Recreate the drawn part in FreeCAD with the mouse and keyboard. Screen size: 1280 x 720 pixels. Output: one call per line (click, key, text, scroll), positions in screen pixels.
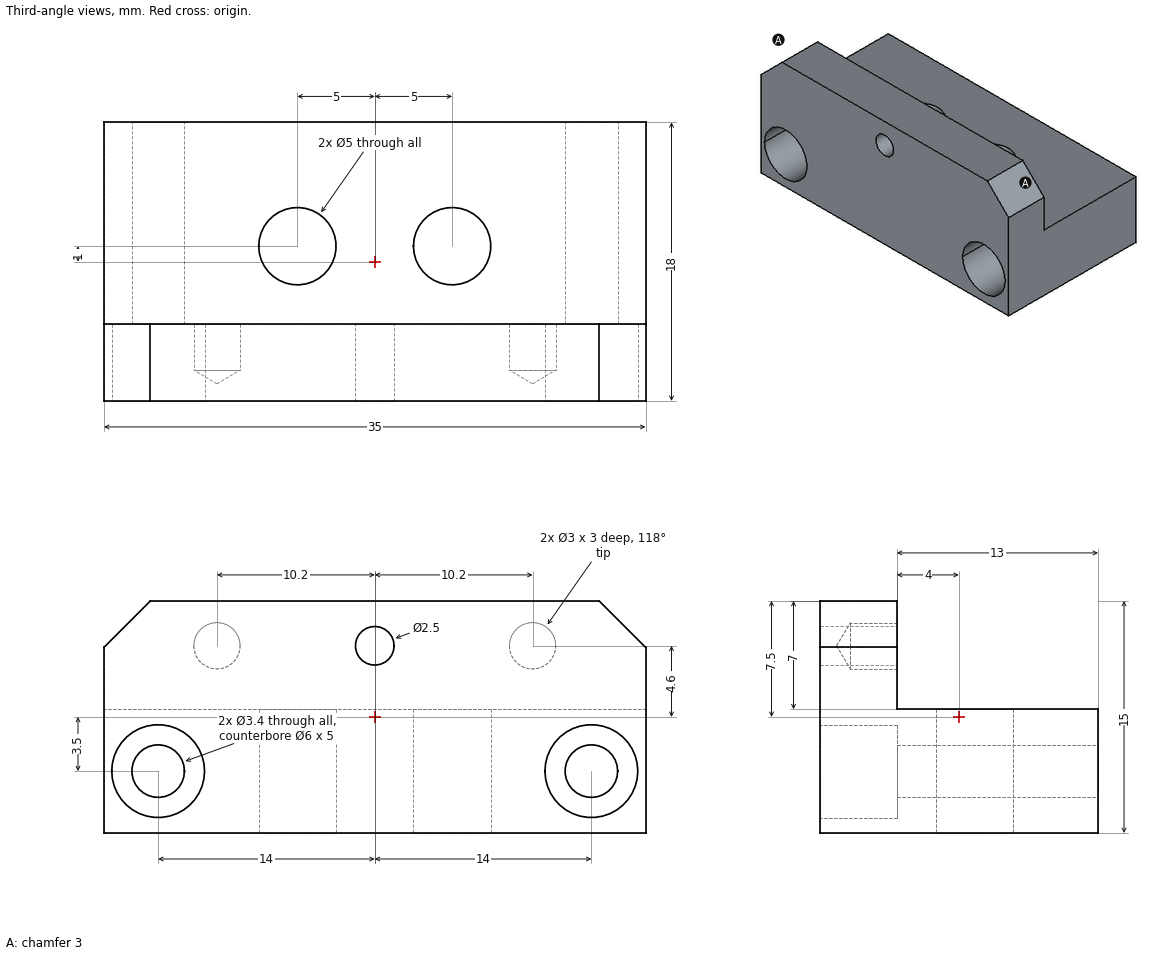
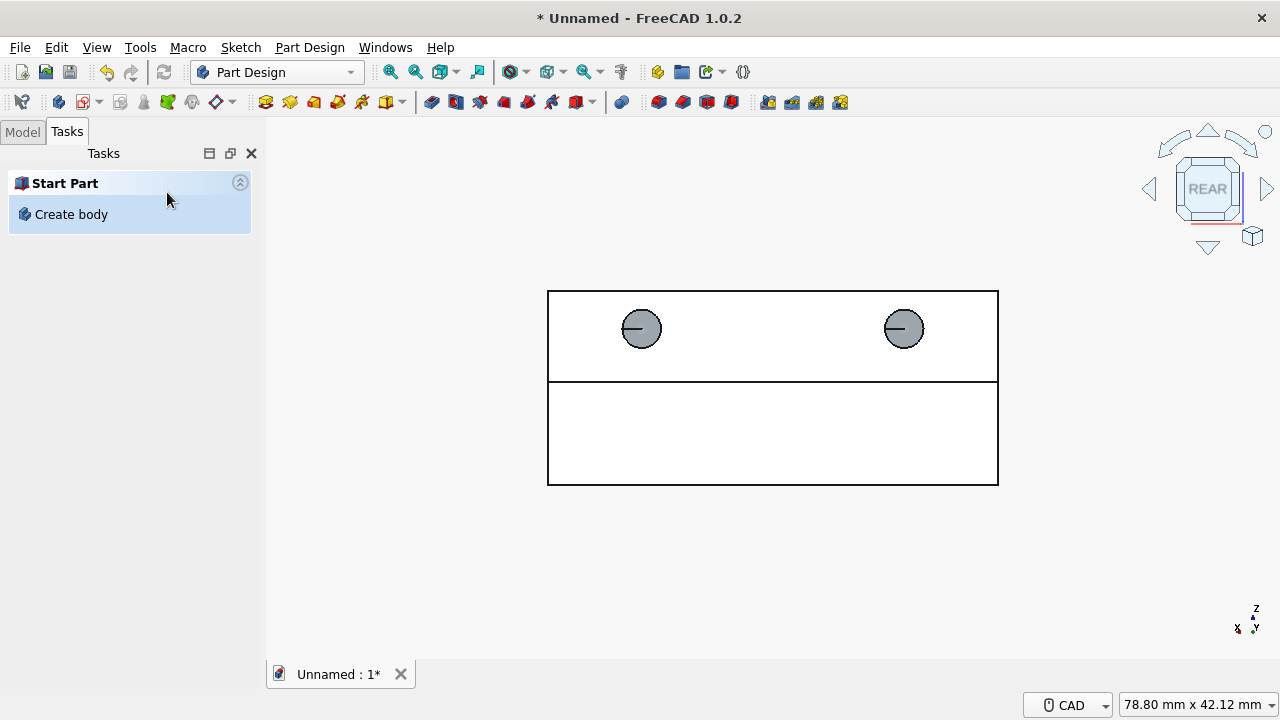
click(392, 72)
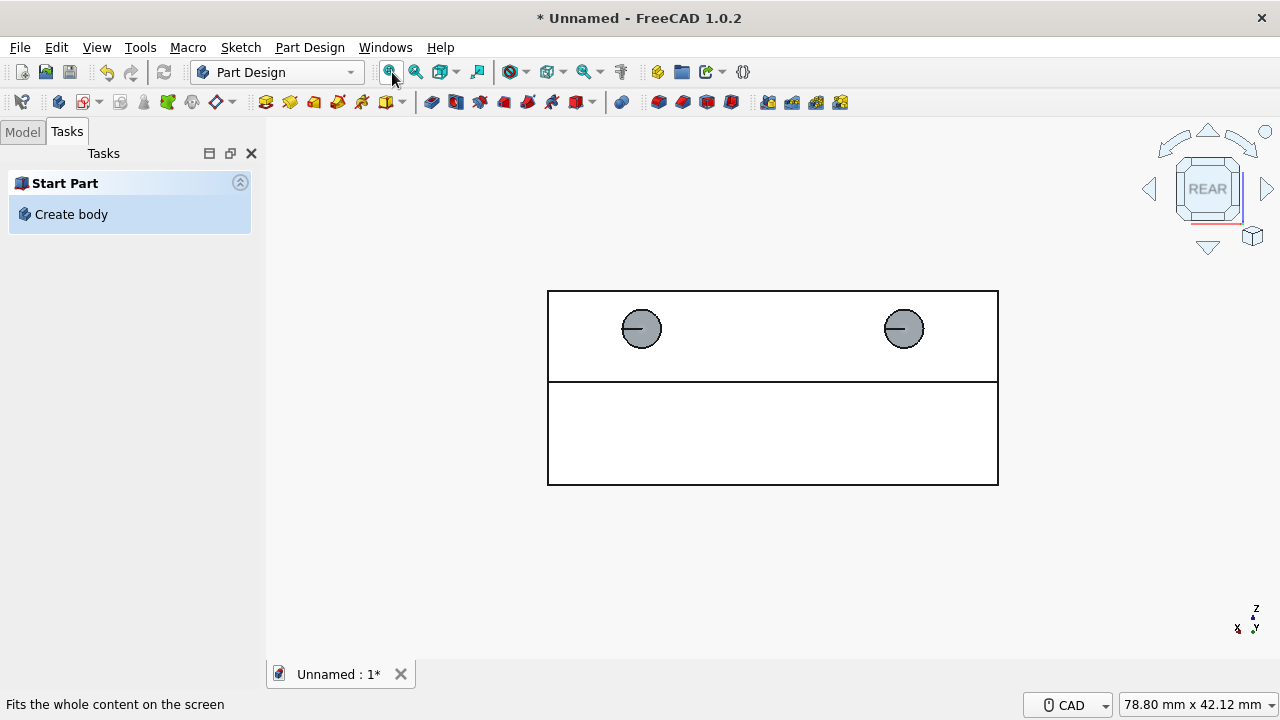
key(0)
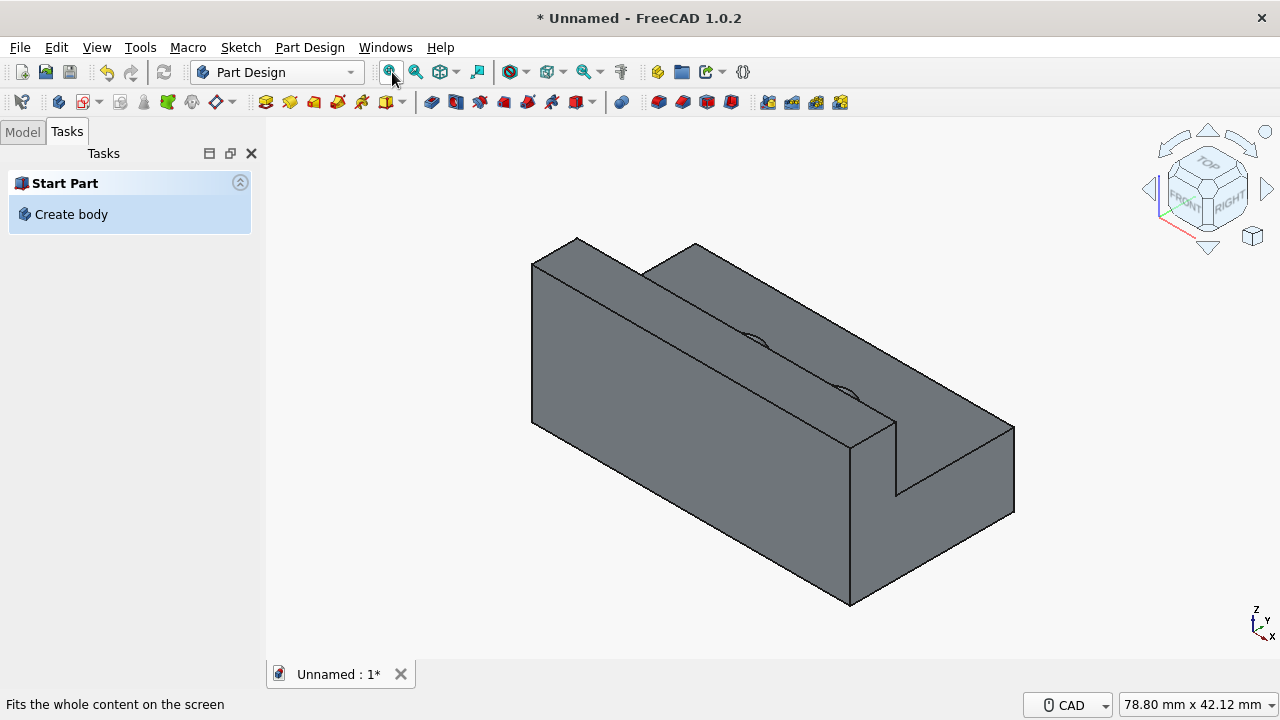
click(782, 487)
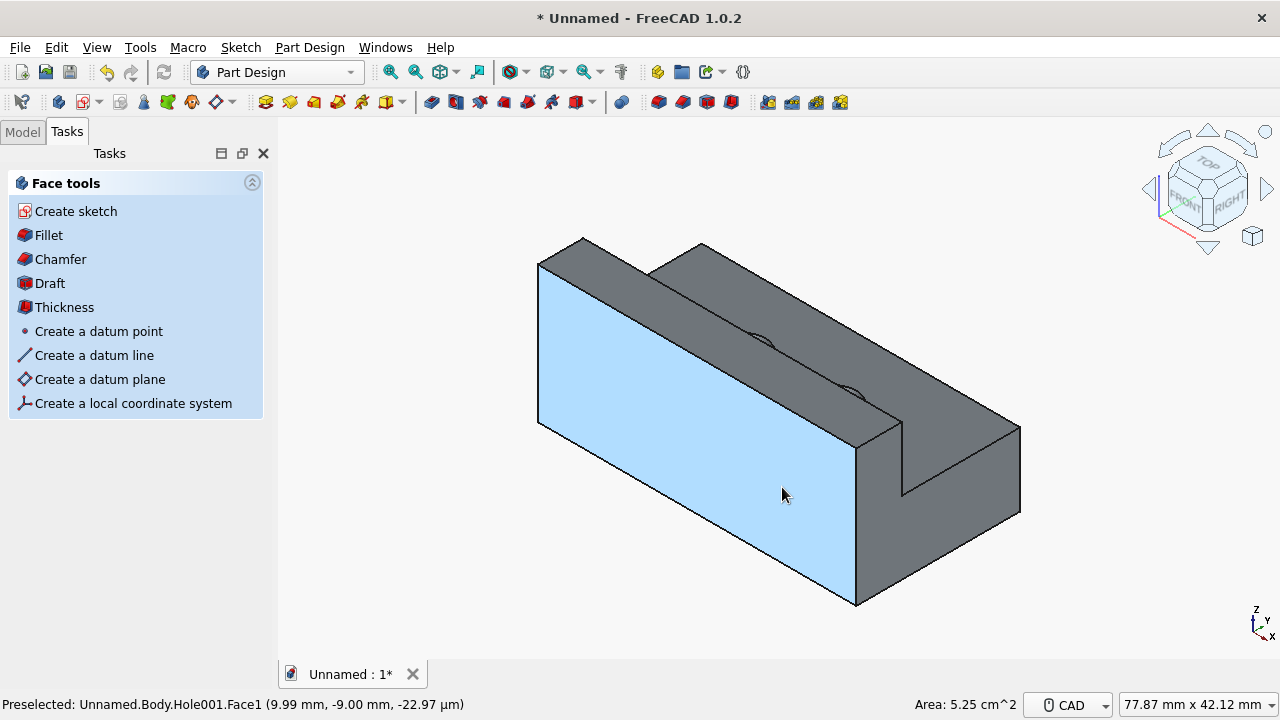
click(84, 102)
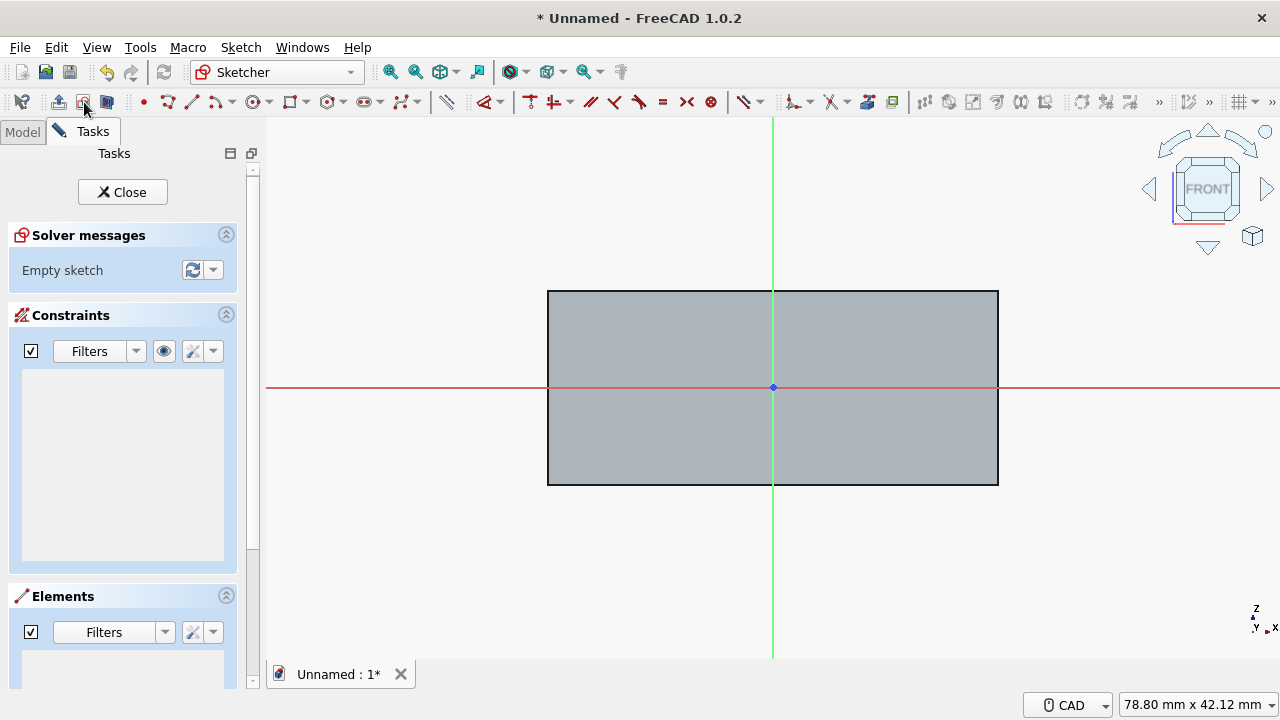
scroll(790, 341, up, 8)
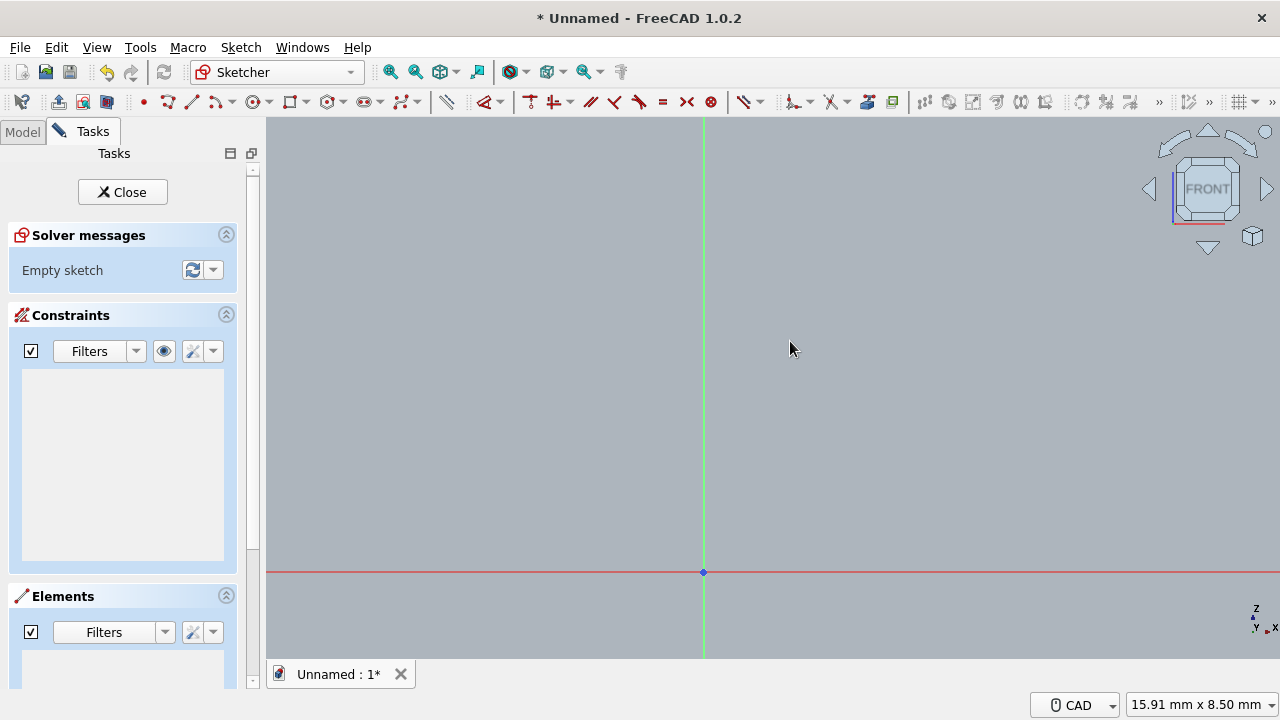
click(254, 102)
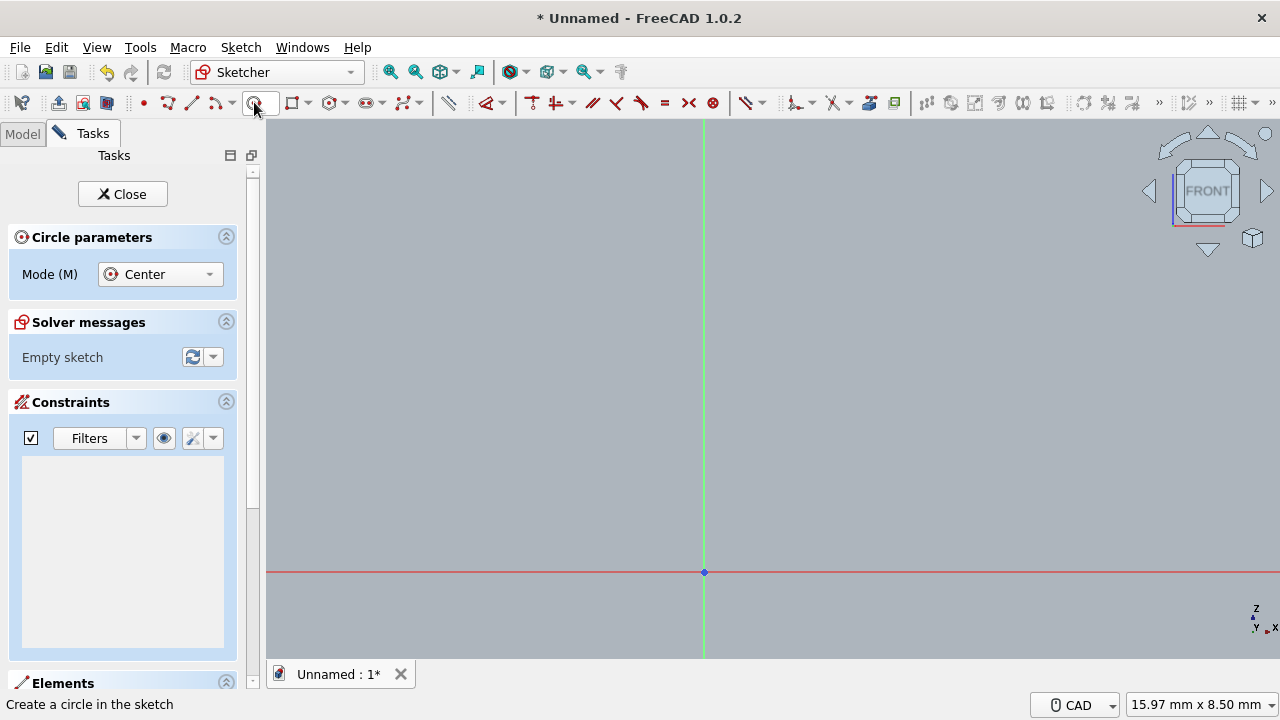
click(704, 280)
click(760, 224)
key(Escape)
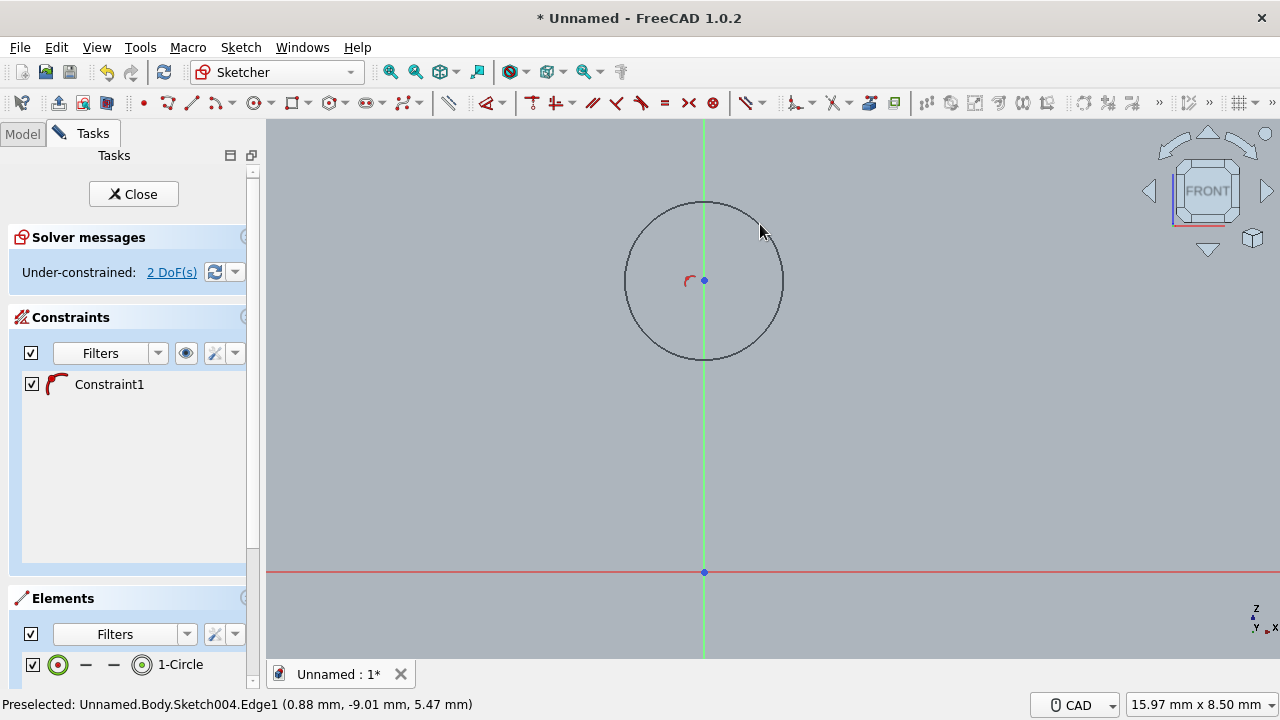
click(486, 104)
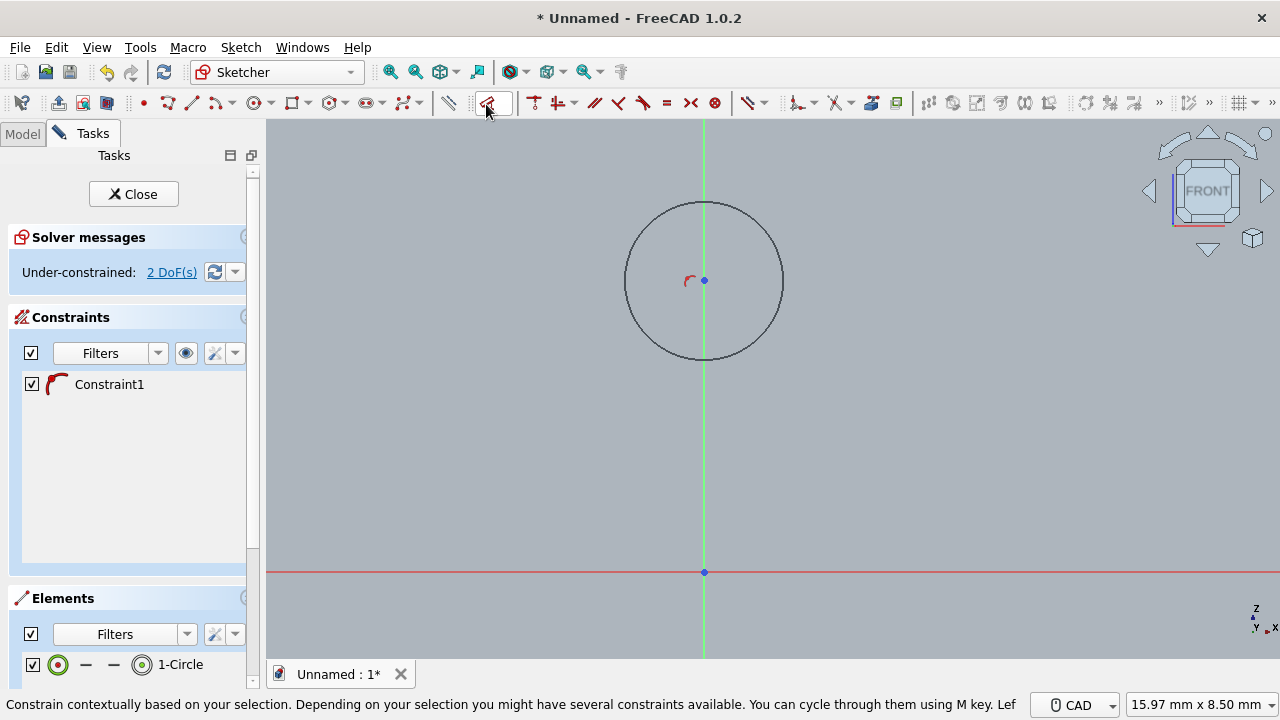
click(760, 225)
click(783, 202)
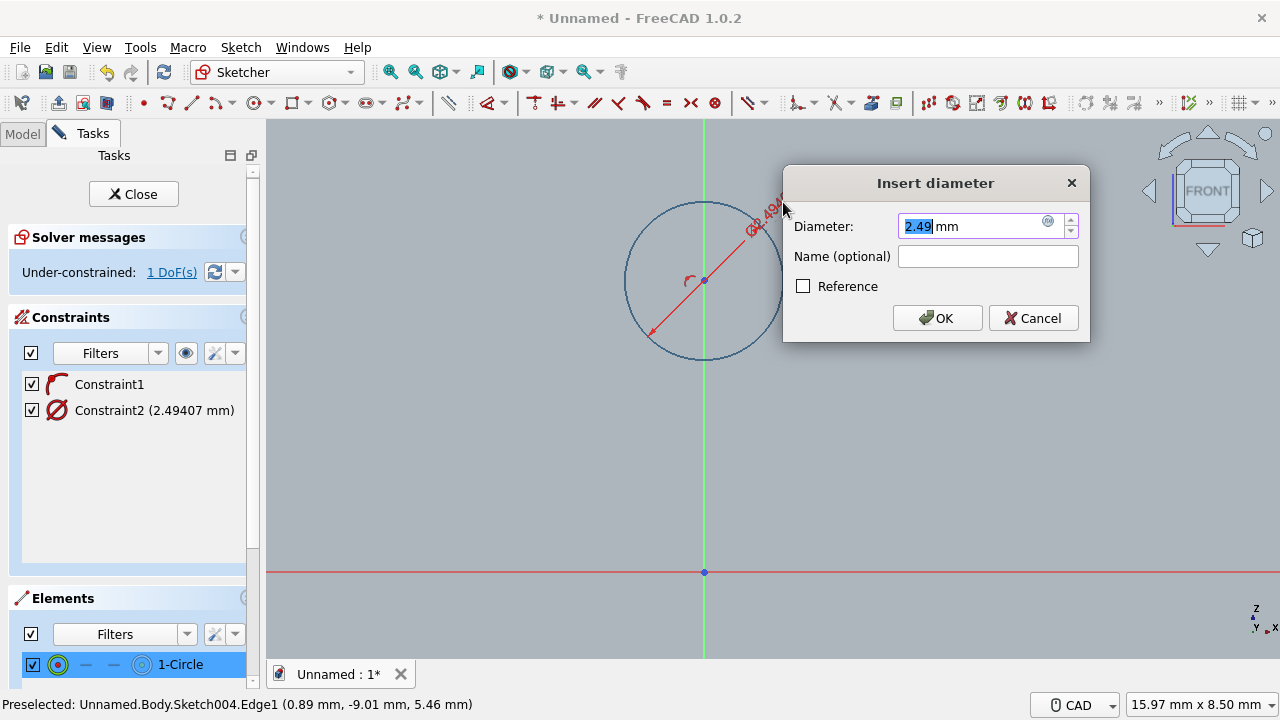
text(2.5)
key(Return)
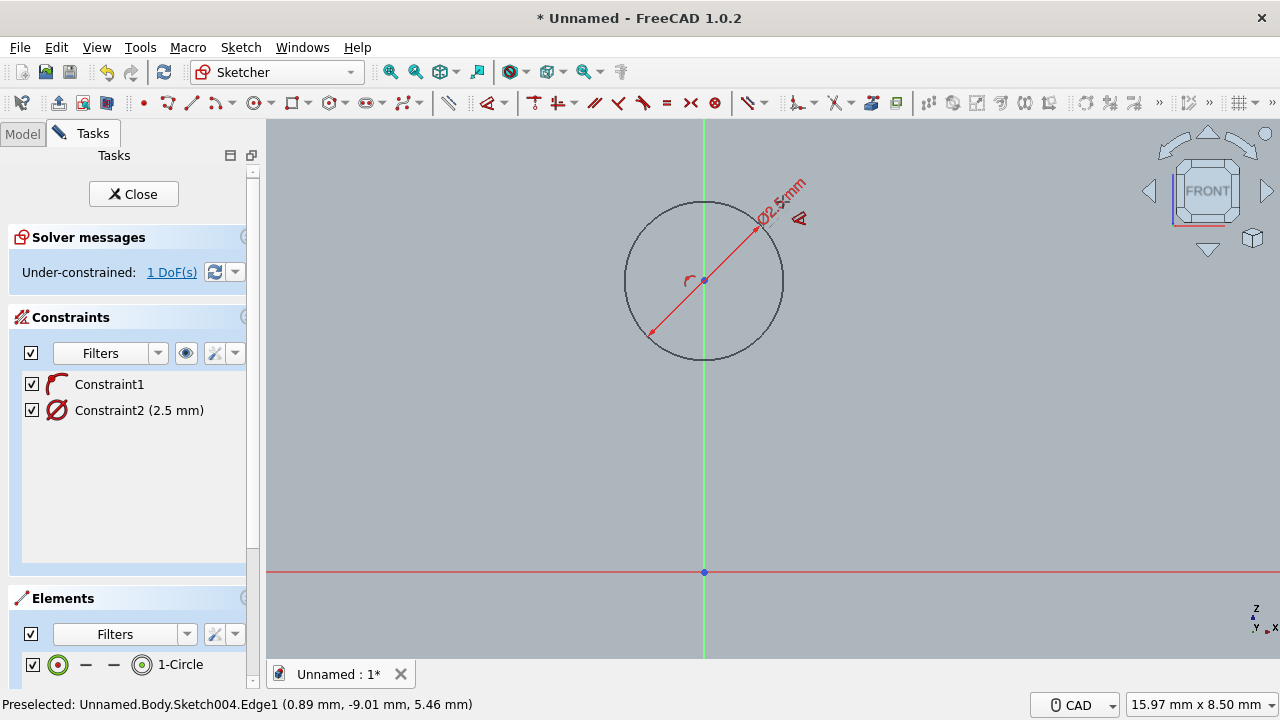
click(704, 281)
click(738, 427)